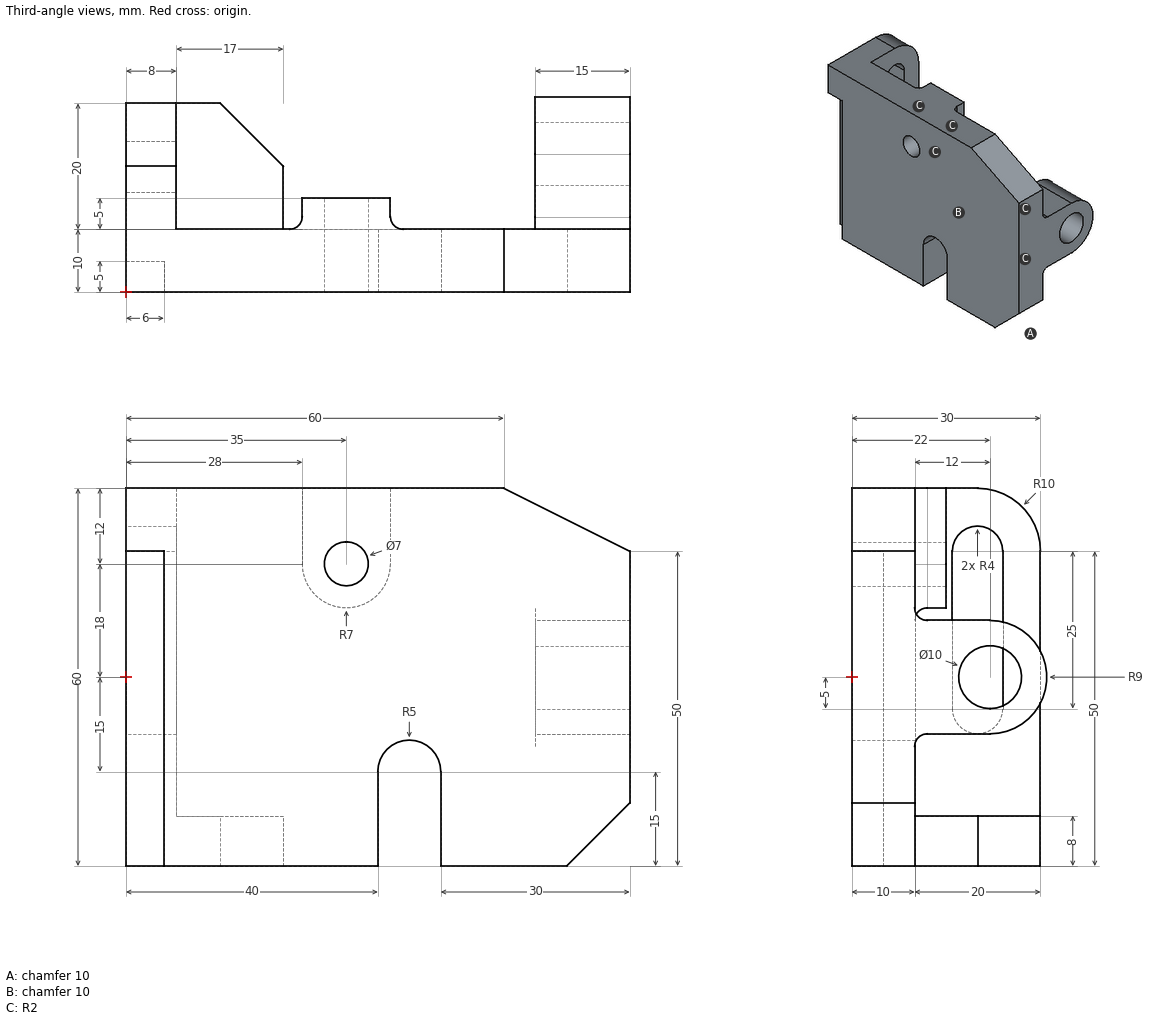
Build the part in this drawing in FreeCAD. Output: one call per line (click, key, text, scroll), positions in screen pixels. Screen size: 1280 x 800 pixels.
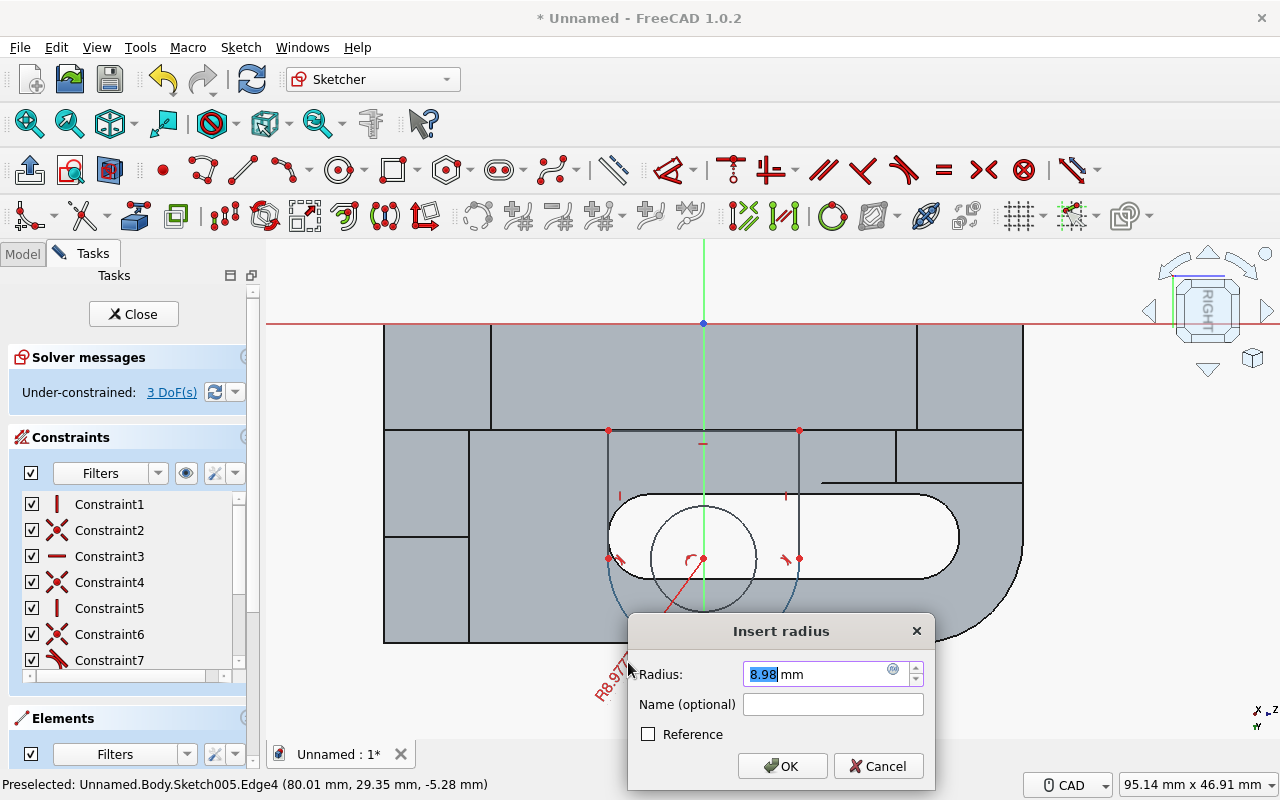
text(9)
key(Return)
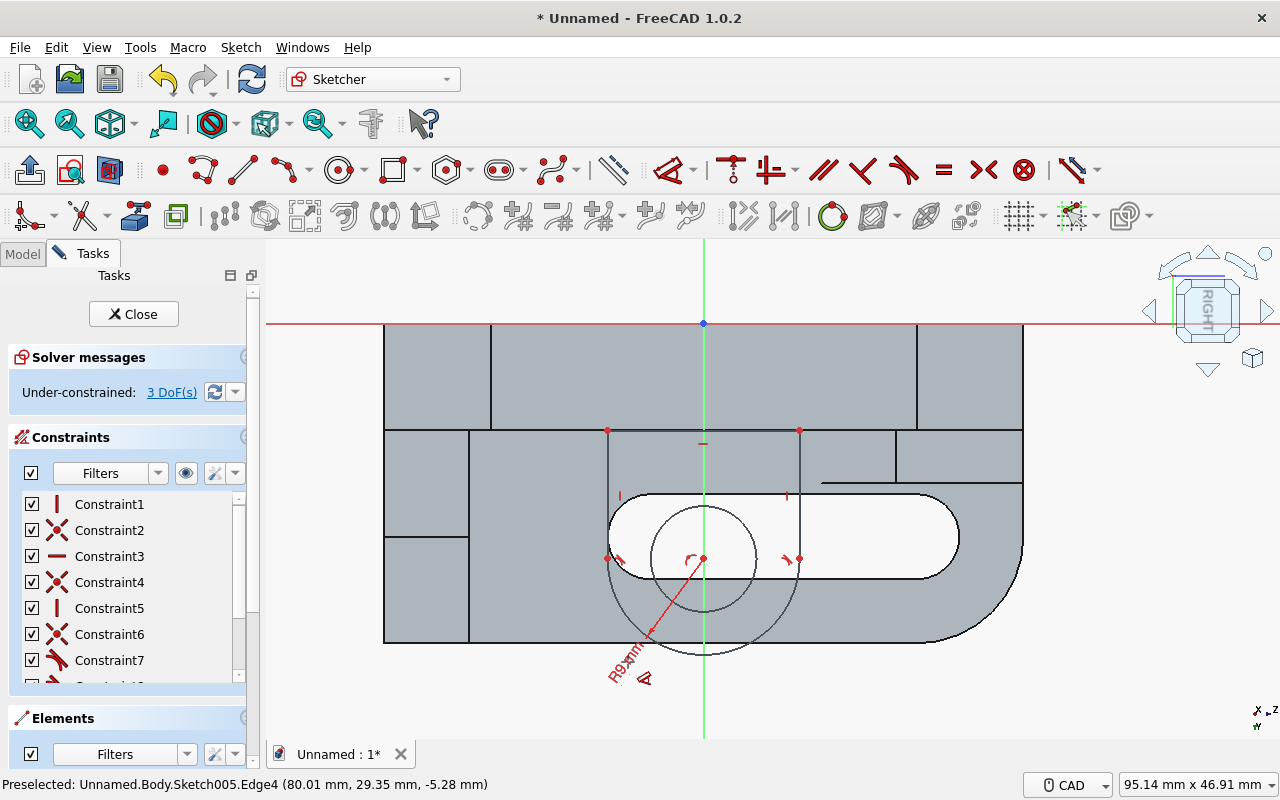
click(741, 521)
click(763, 498)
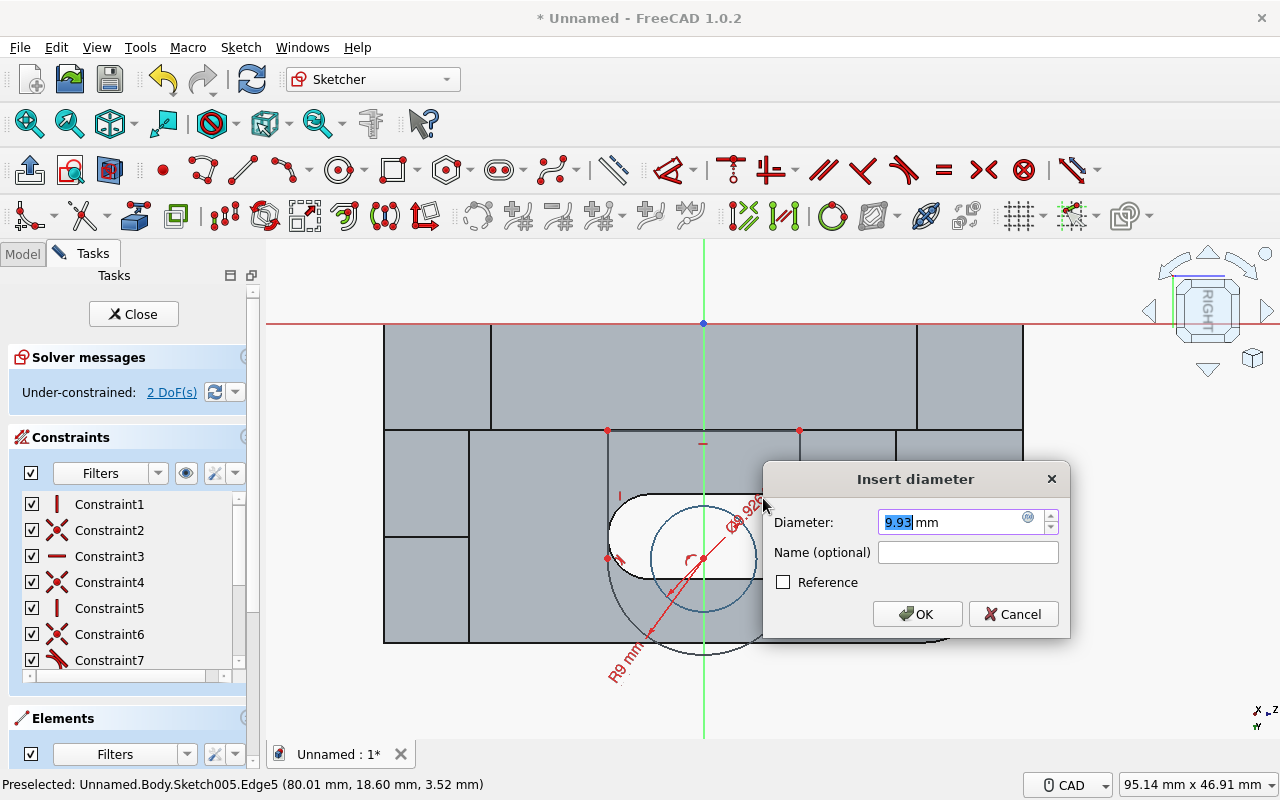
text(10)
key(Return)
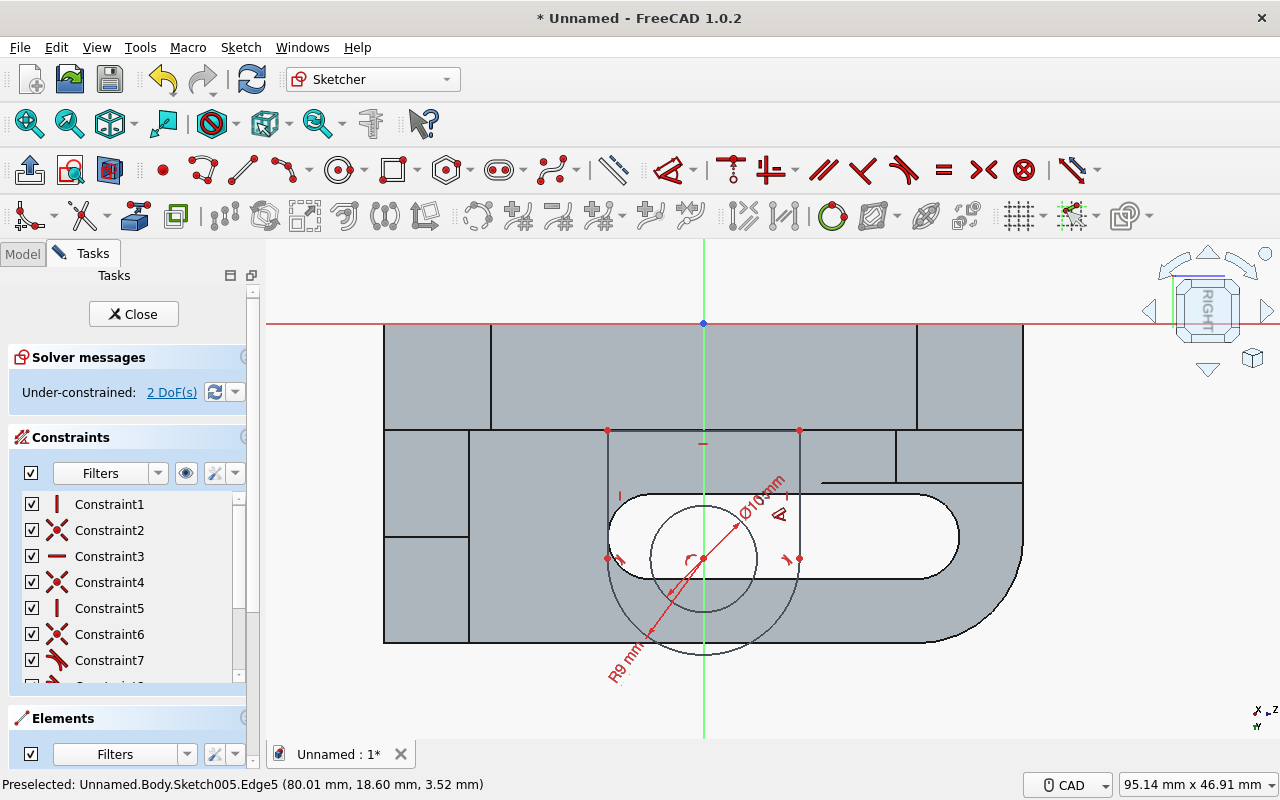
click(800, 521)
click(834, 495)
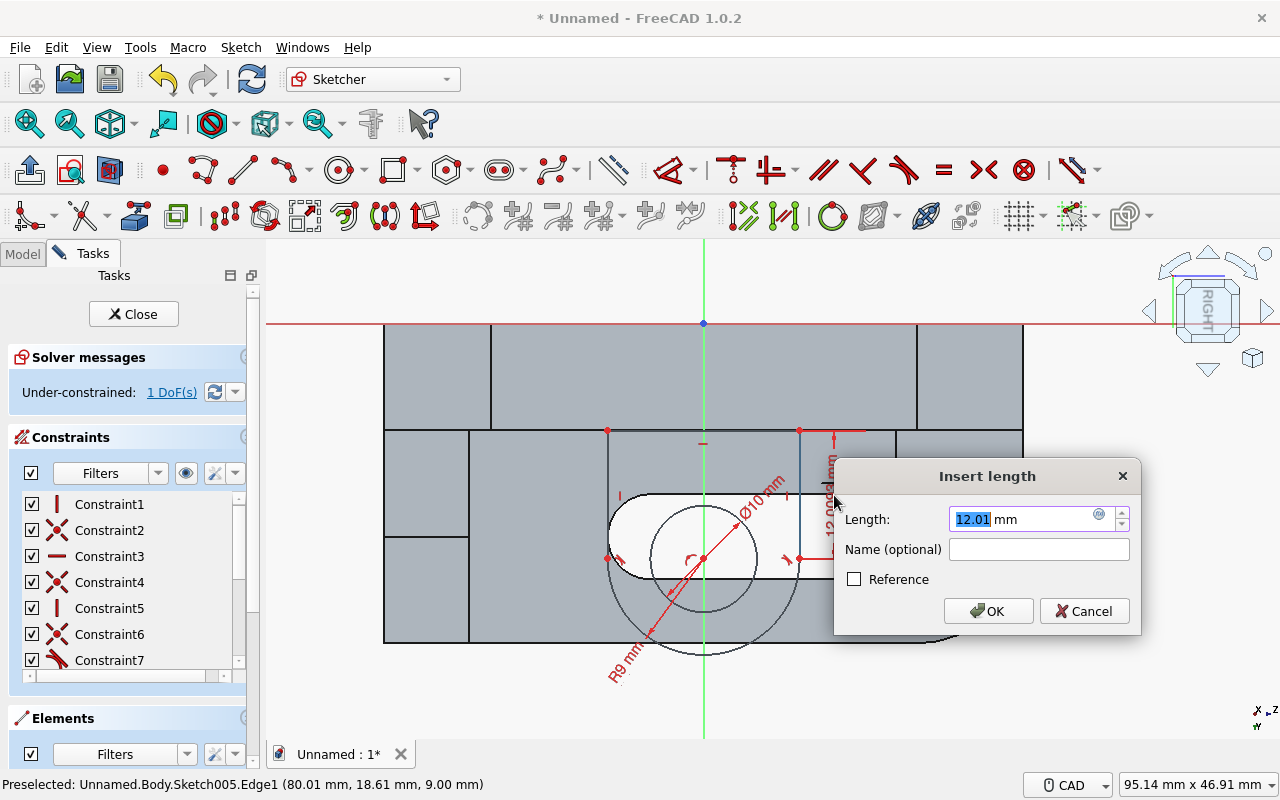
text(12)
key(Return)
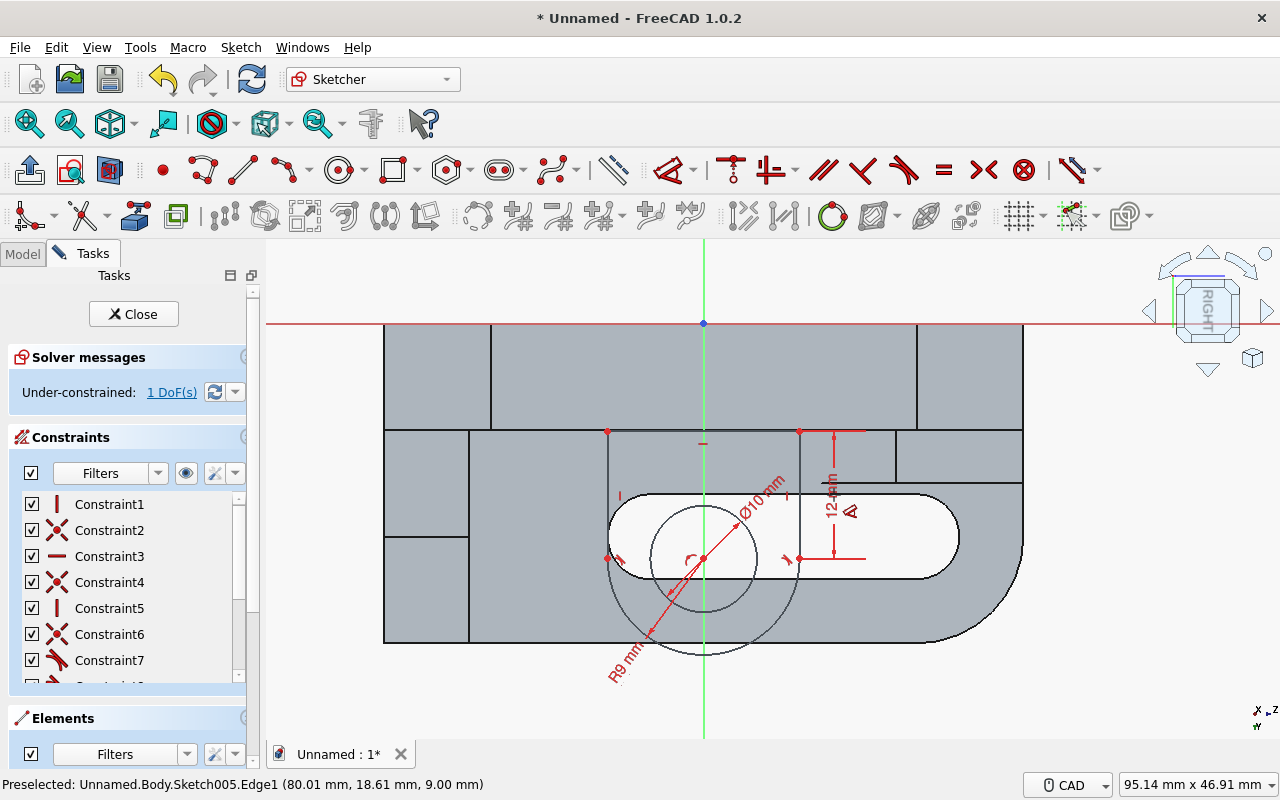
click(704, 559)
click(738, 387)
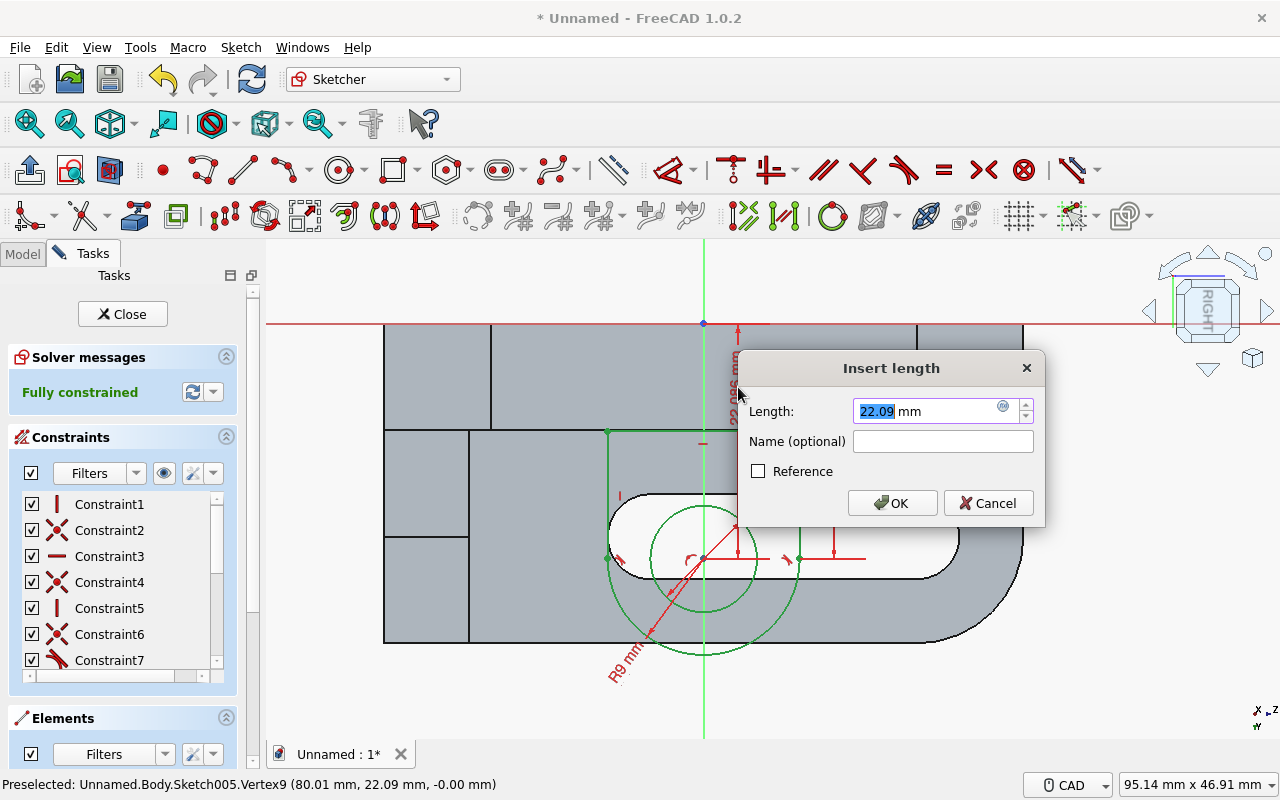
text(22)
key(Return)
key(Escape)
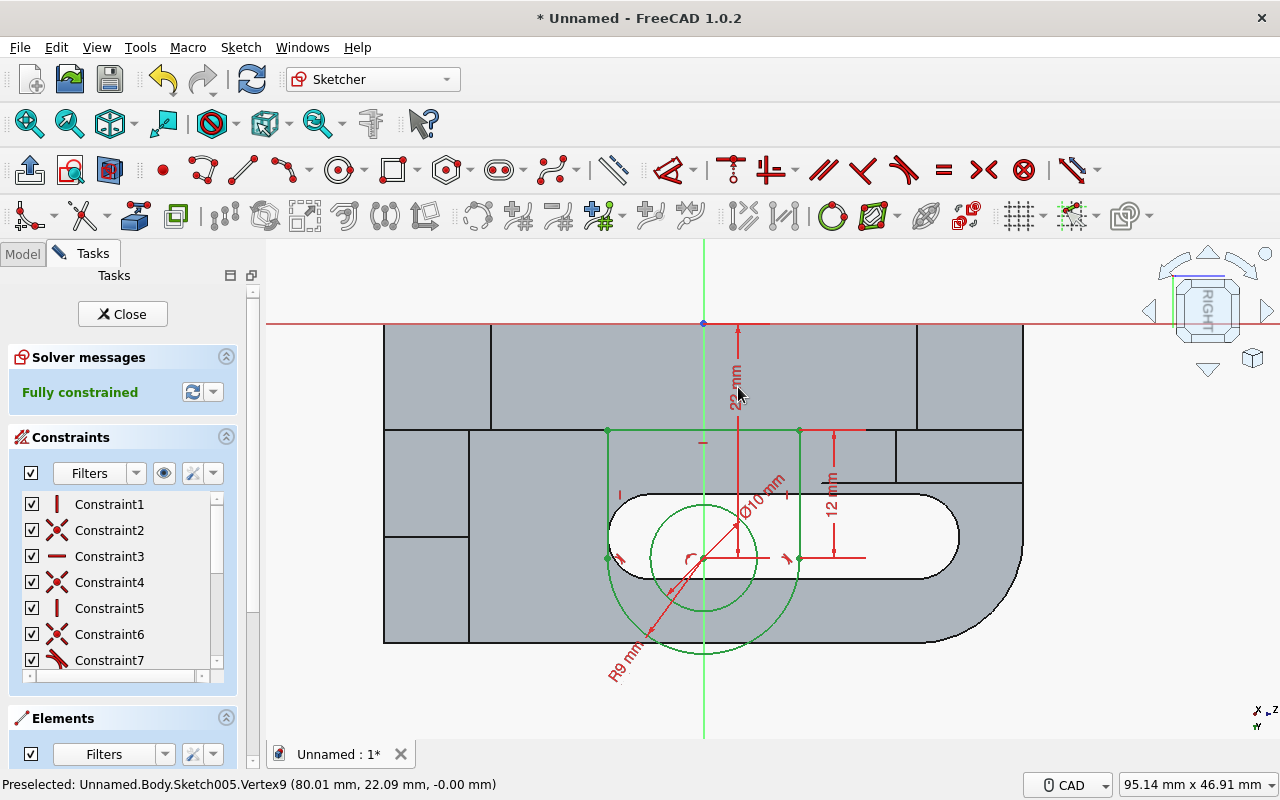
click(123, 314)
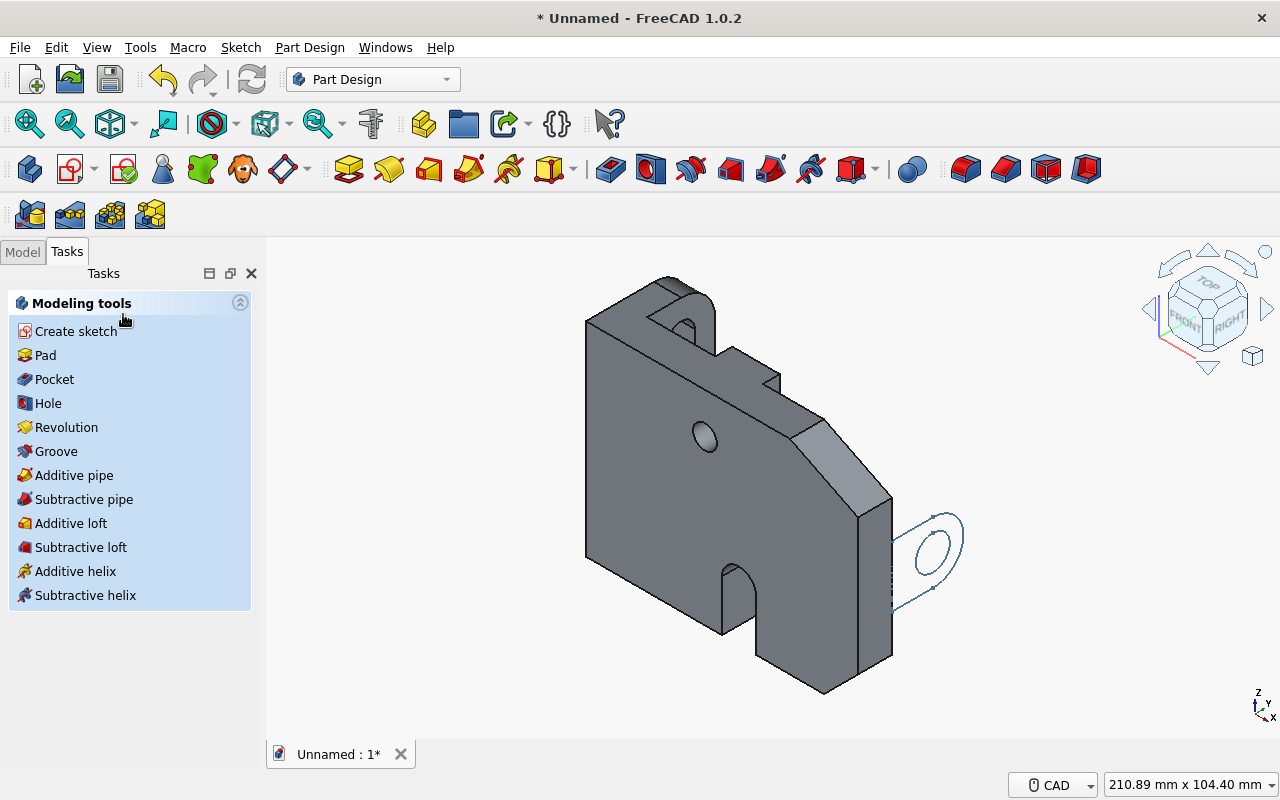
click(350, 170)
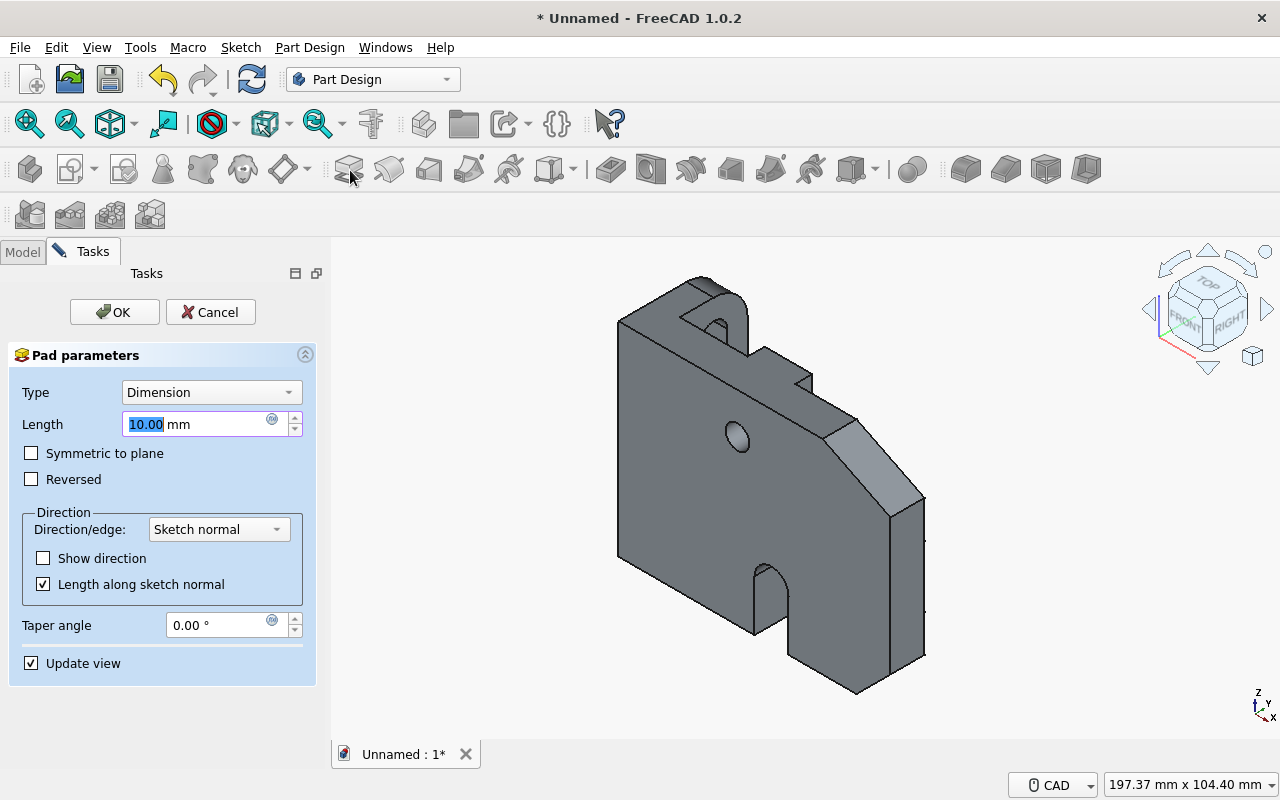
text(15)
key(Tab)